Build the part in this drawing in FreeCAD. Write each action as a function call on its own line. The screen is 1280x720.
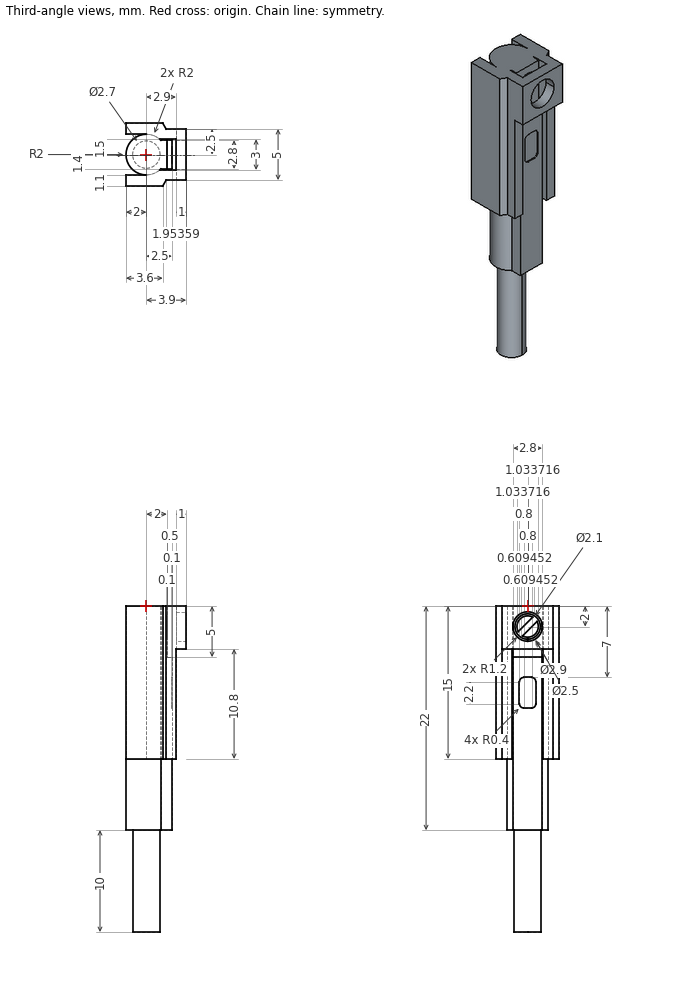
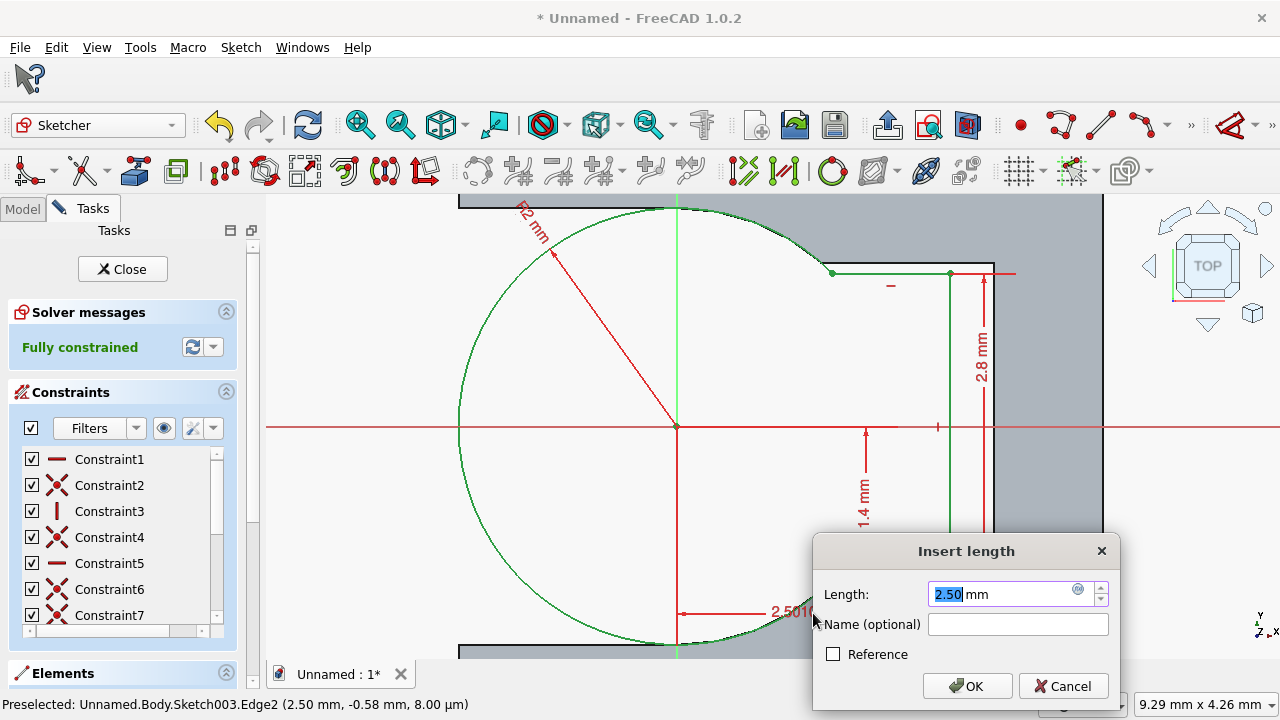
text(2.5)
key(Return)
key(Escape)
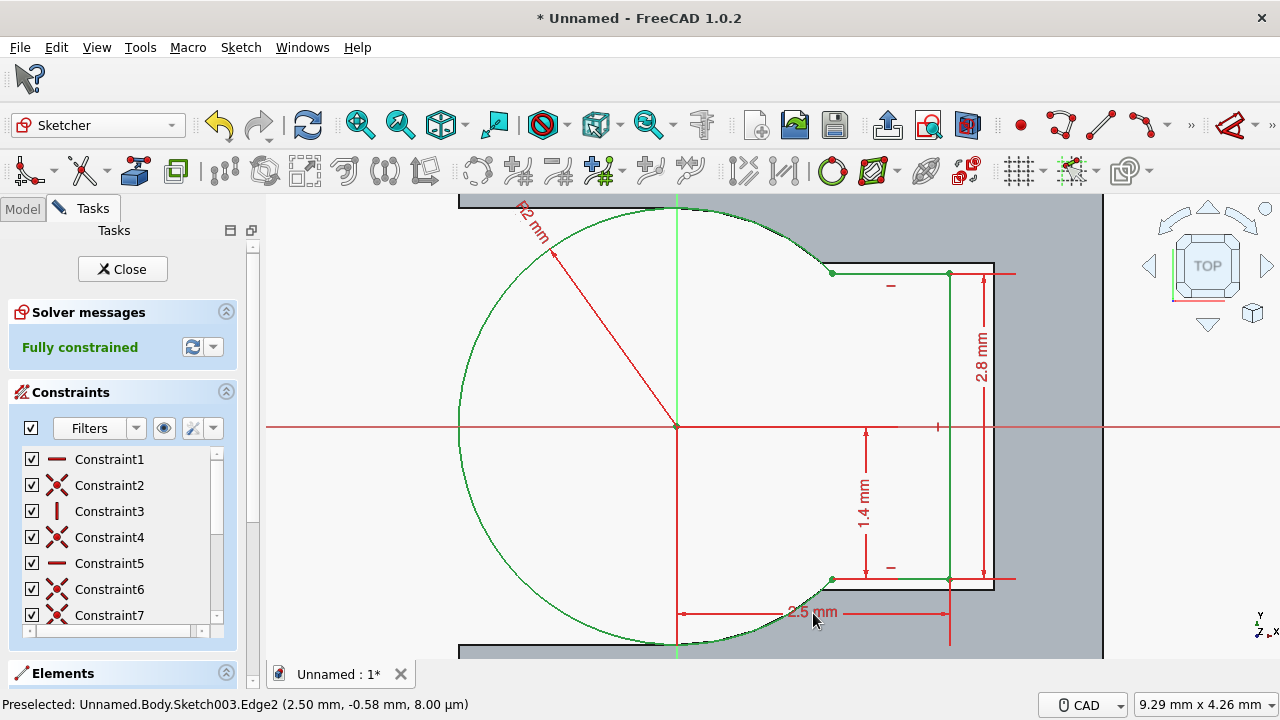
click(123, 269)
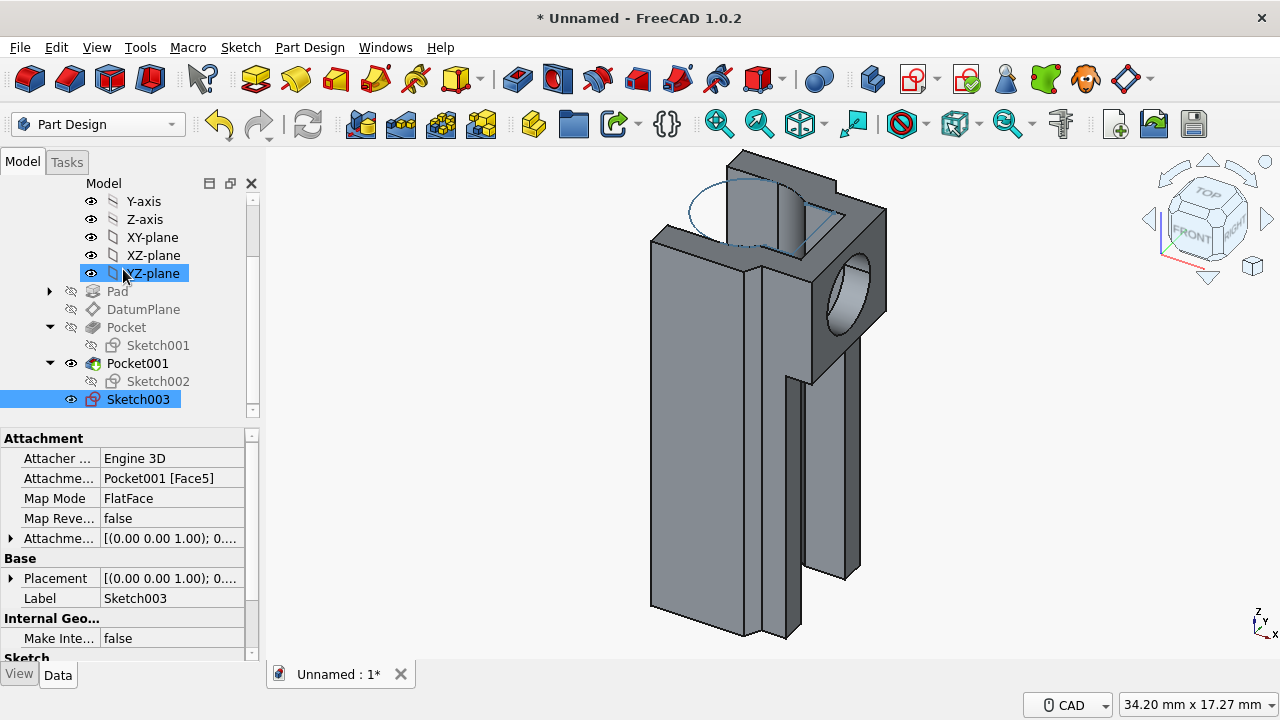
click(256, 80)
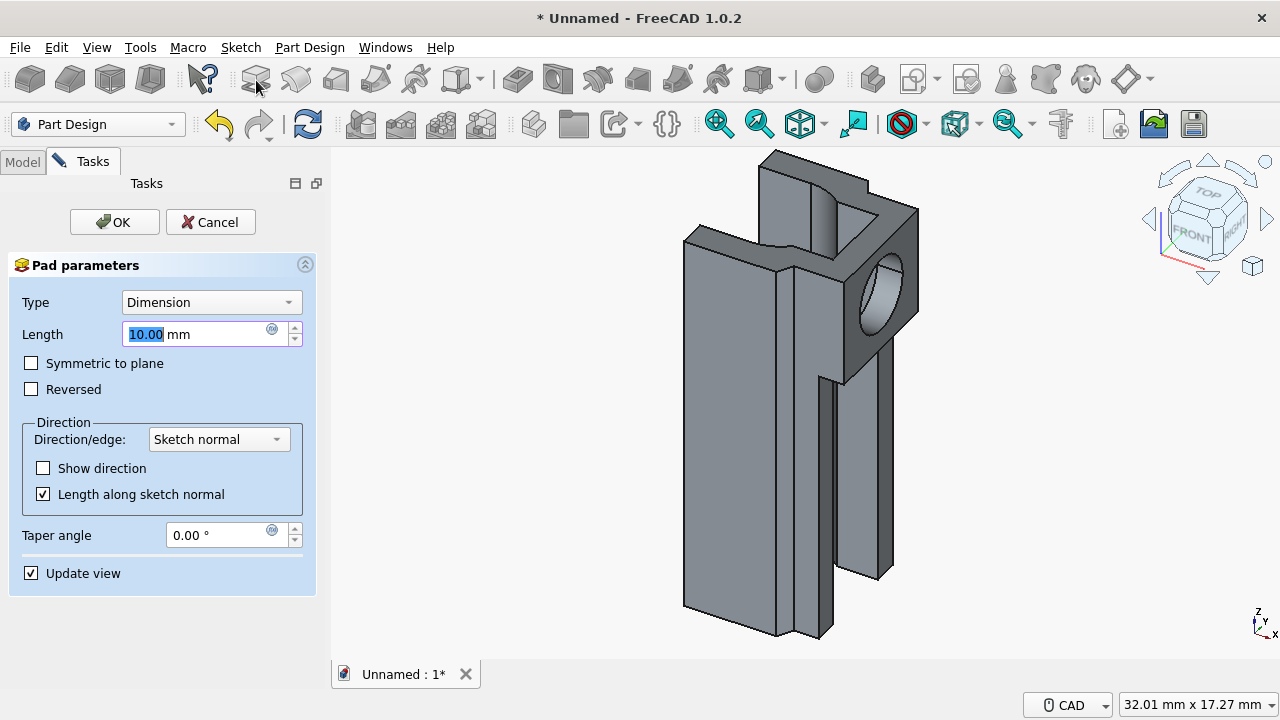
text(22)
key(Tab)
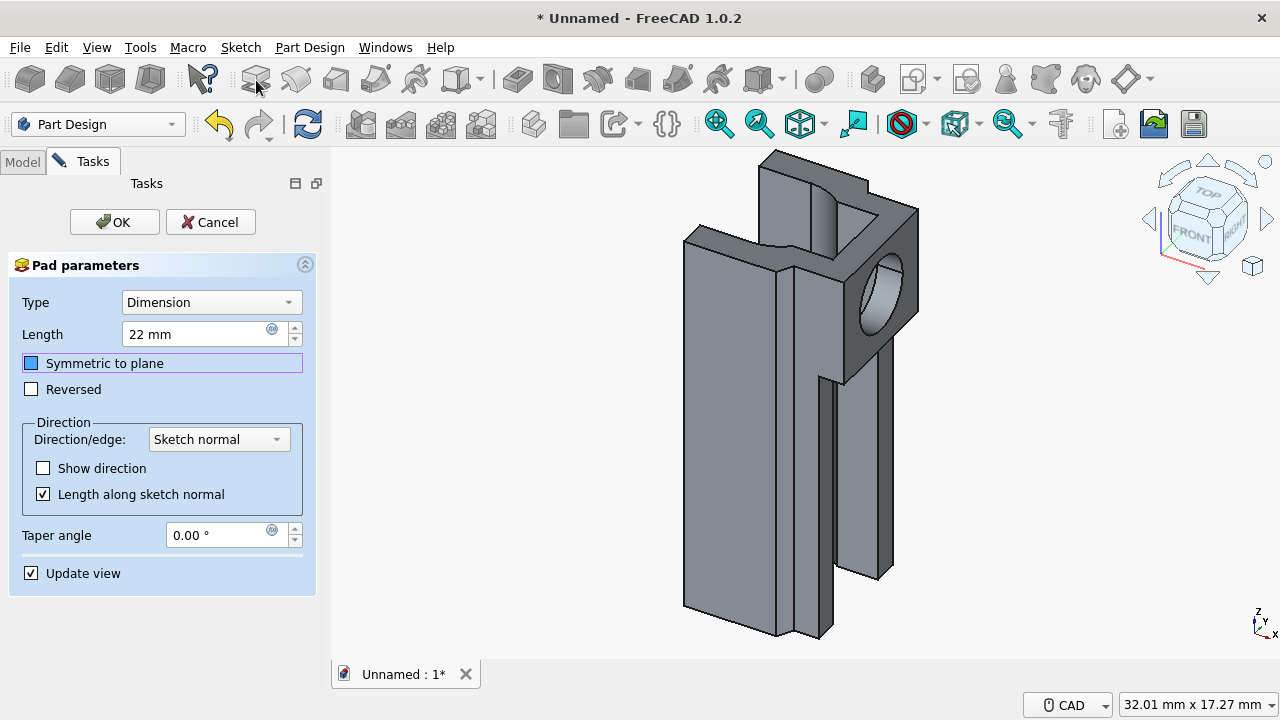
click(30, 389)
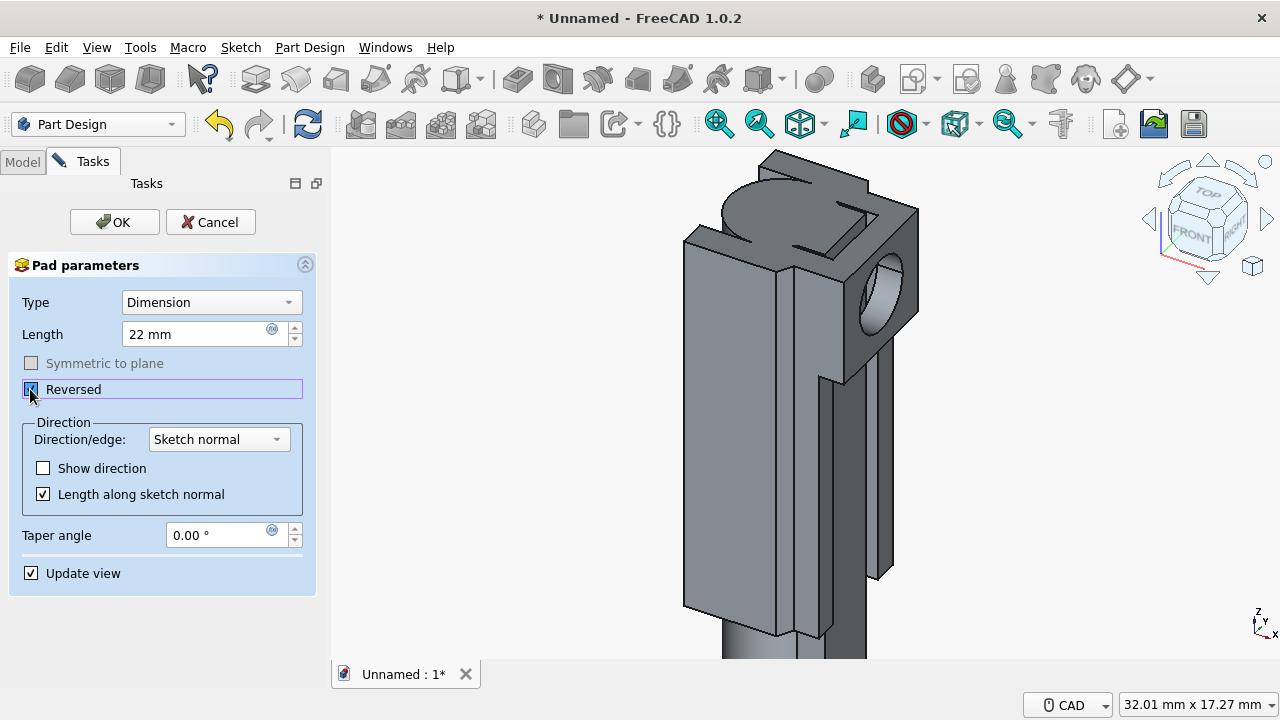
click(115, 222)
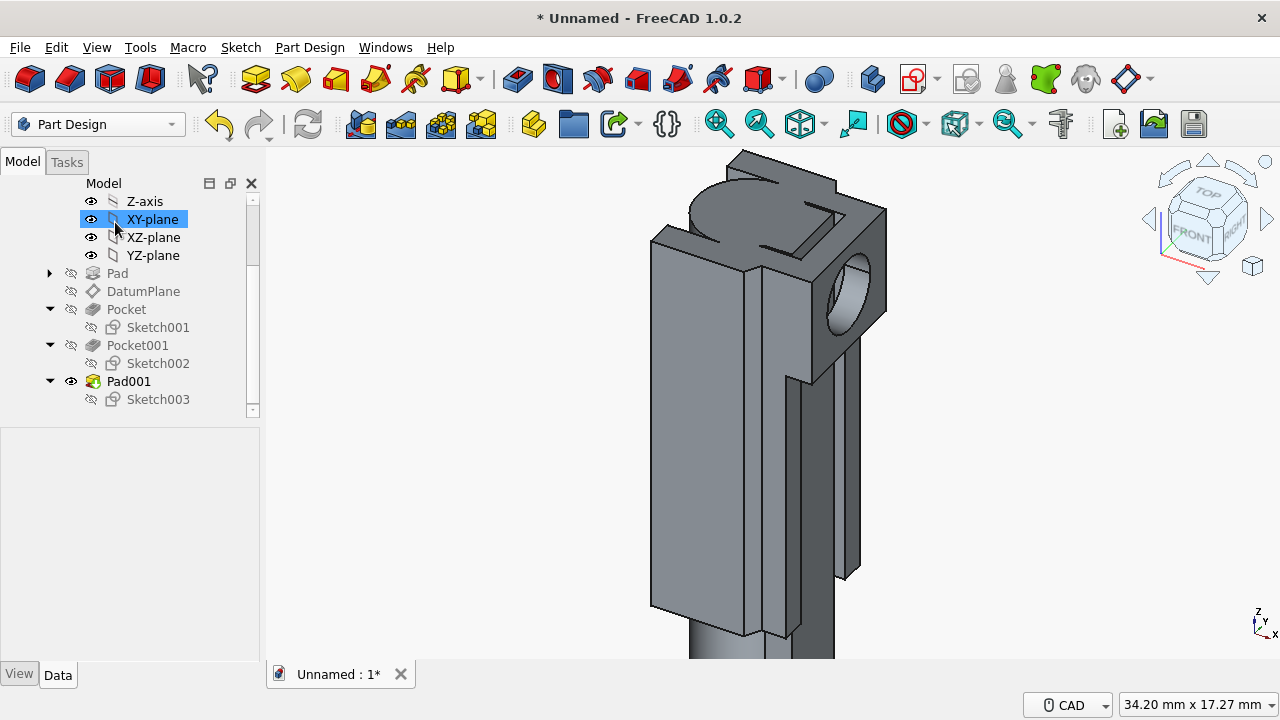
click(720, 124)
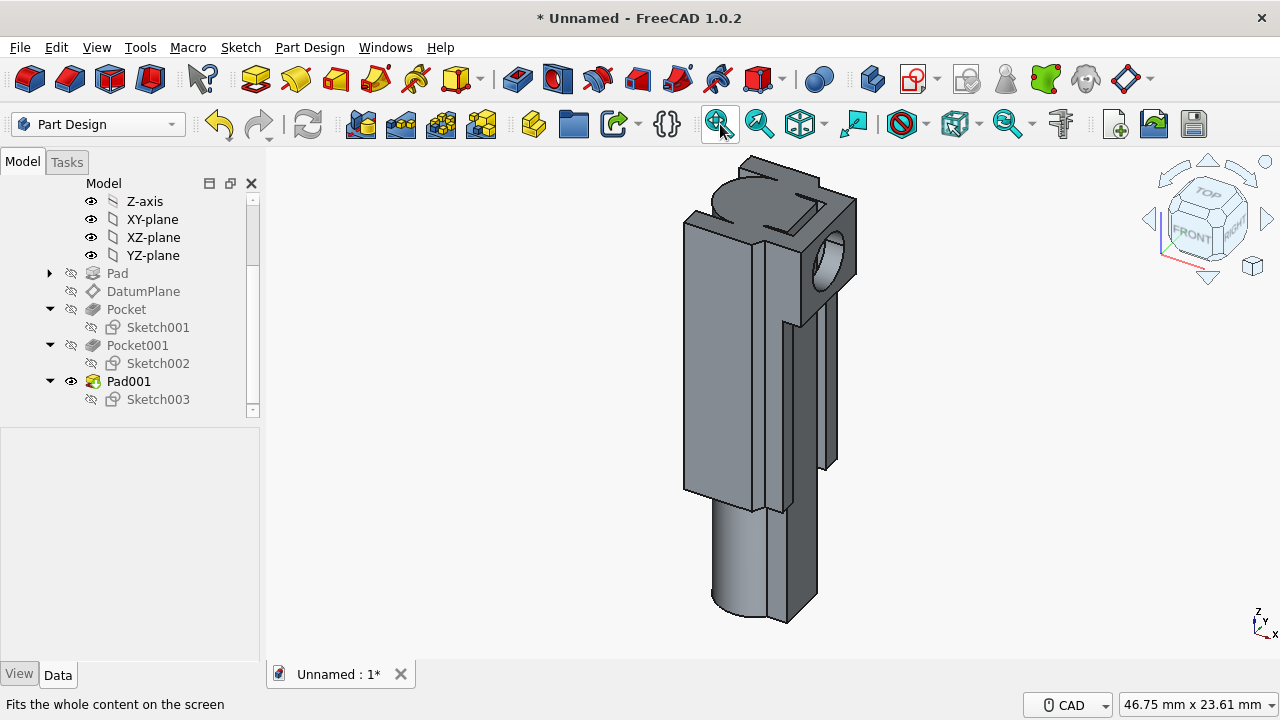
click(914, 80)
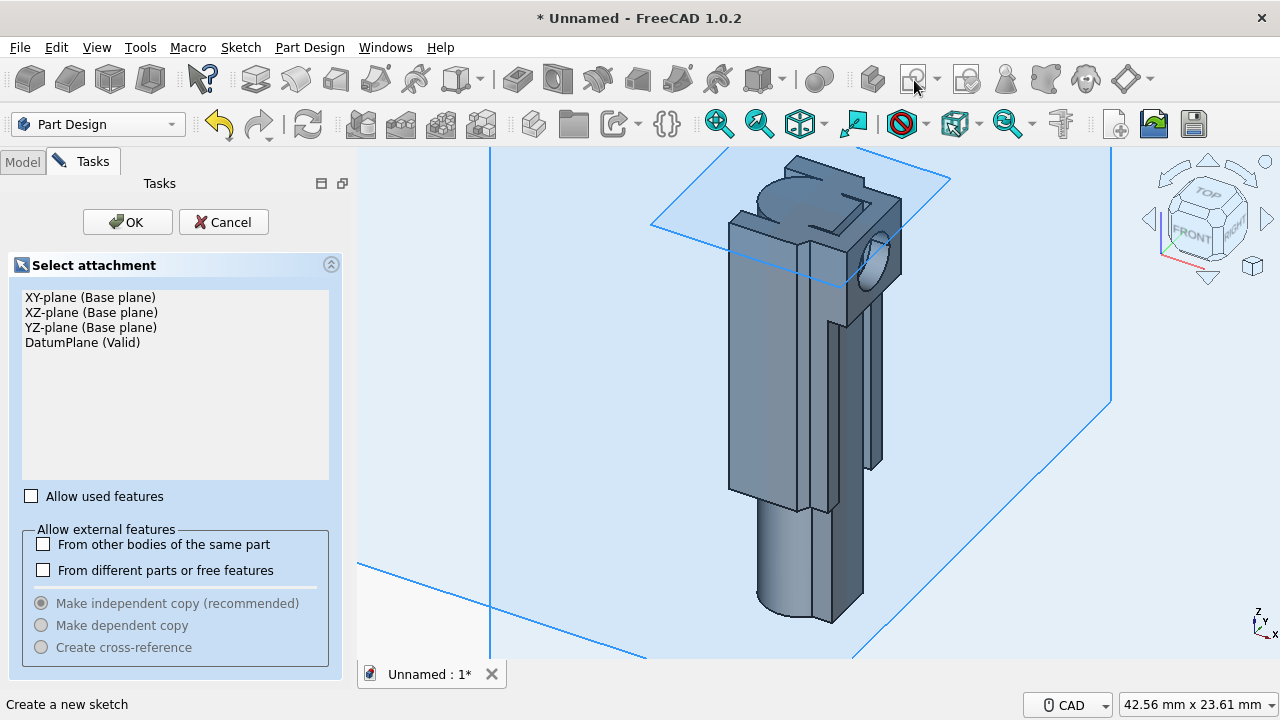
click(82, 312)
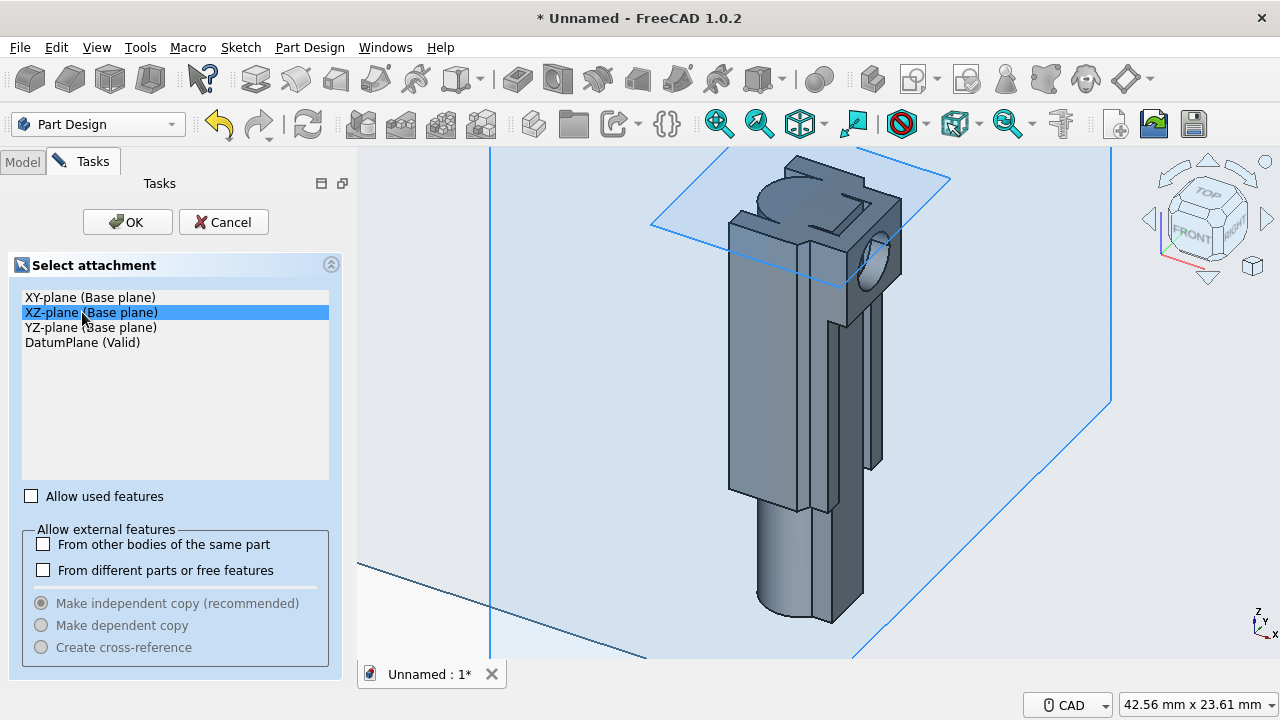
click(128, 222)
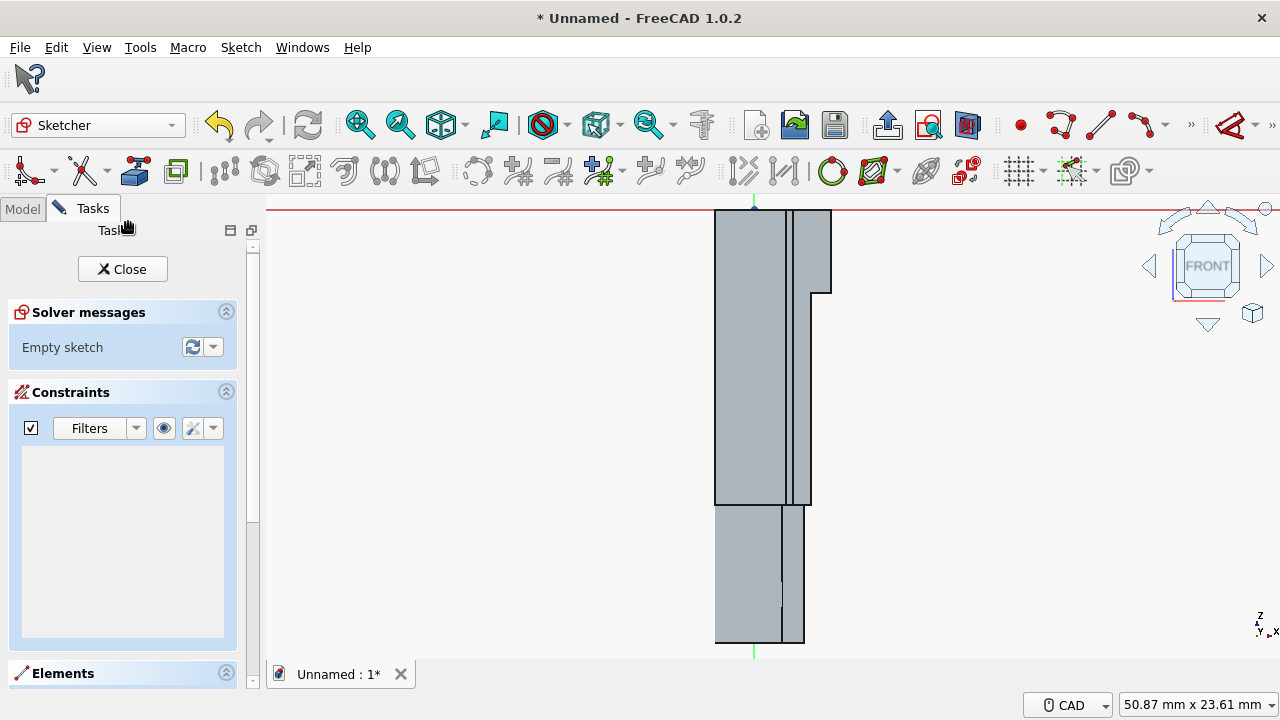
click(968, 126)